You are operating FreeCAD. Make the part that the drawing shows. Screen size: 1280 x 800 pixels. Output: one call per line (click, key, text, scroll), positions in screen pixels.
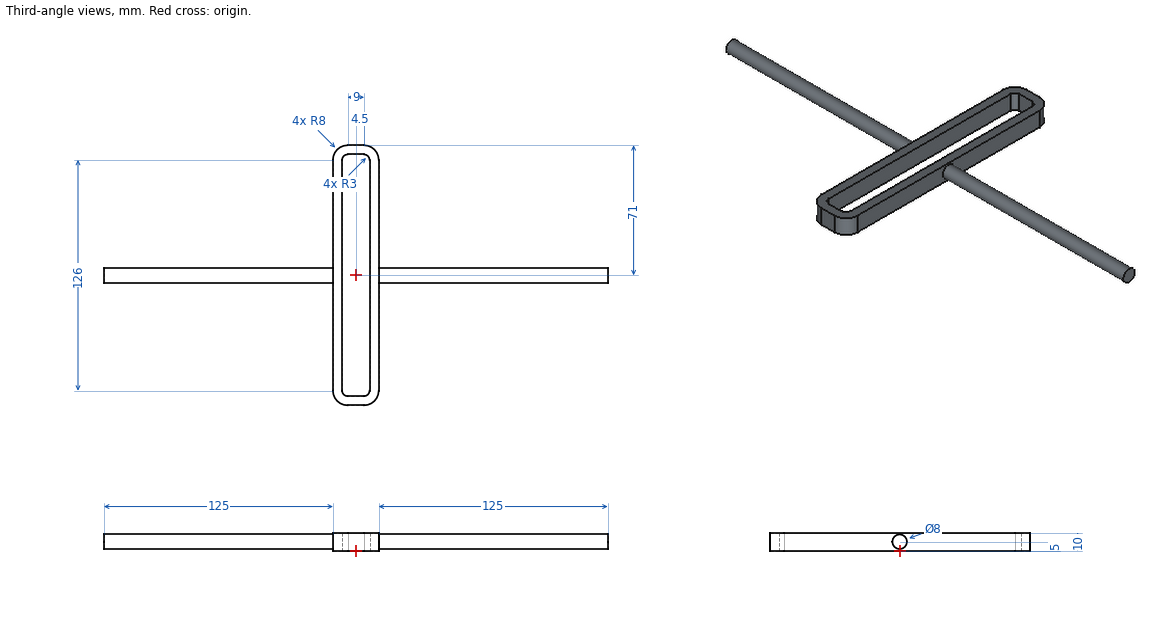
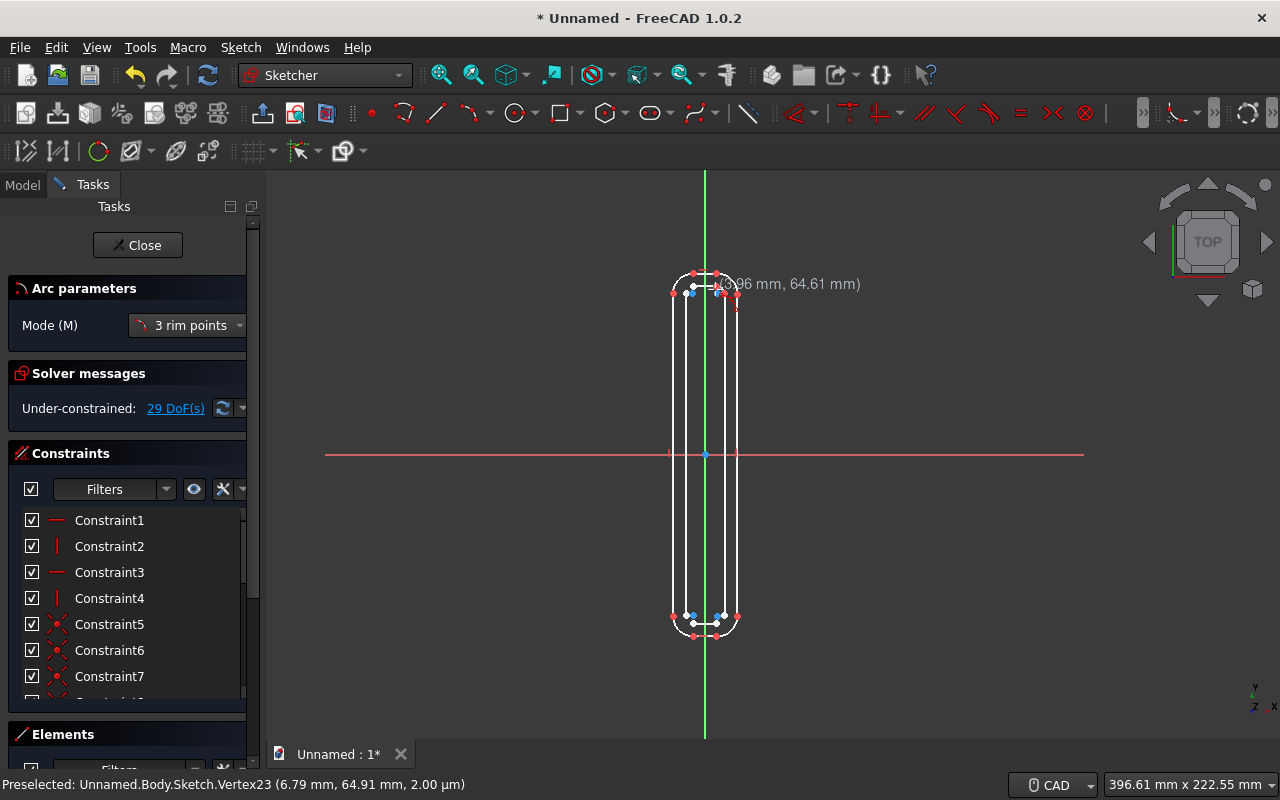
scroll(724, 616, up, 4)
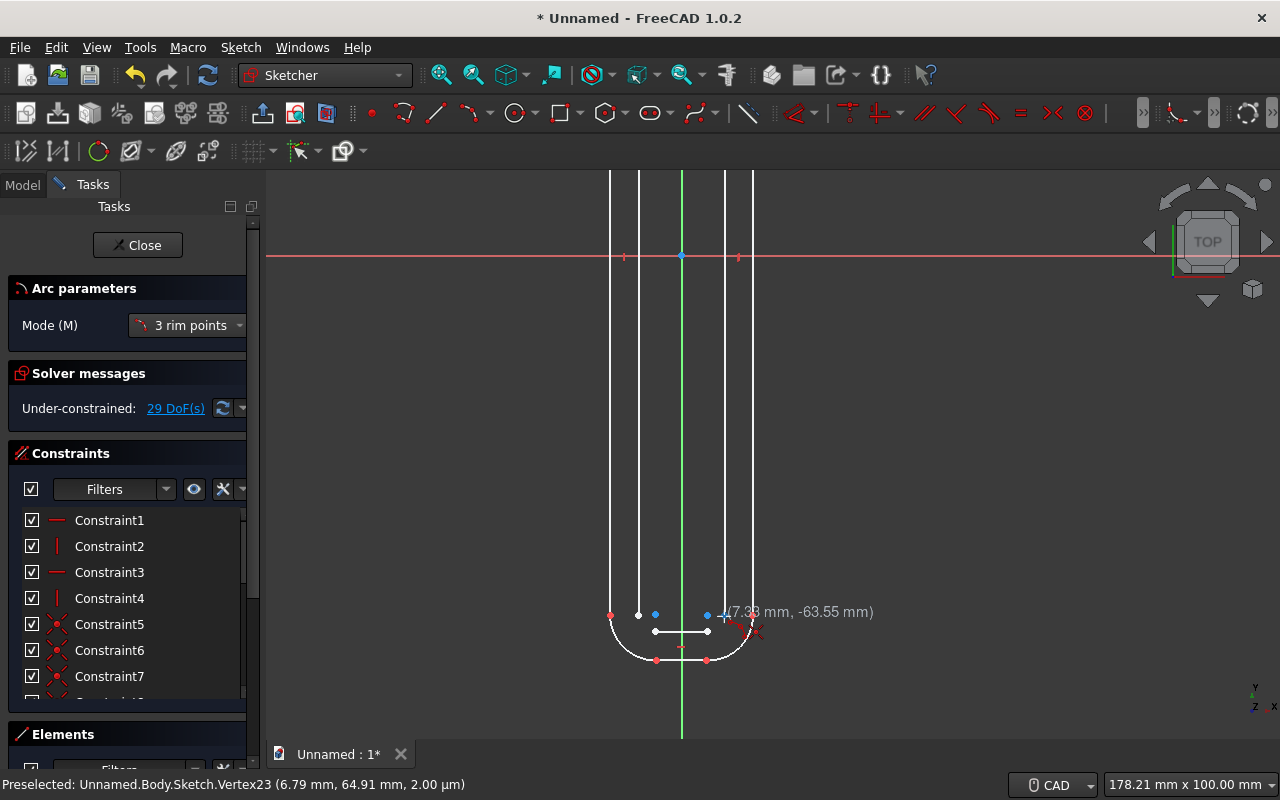
click(725, 615)
click(708, 632)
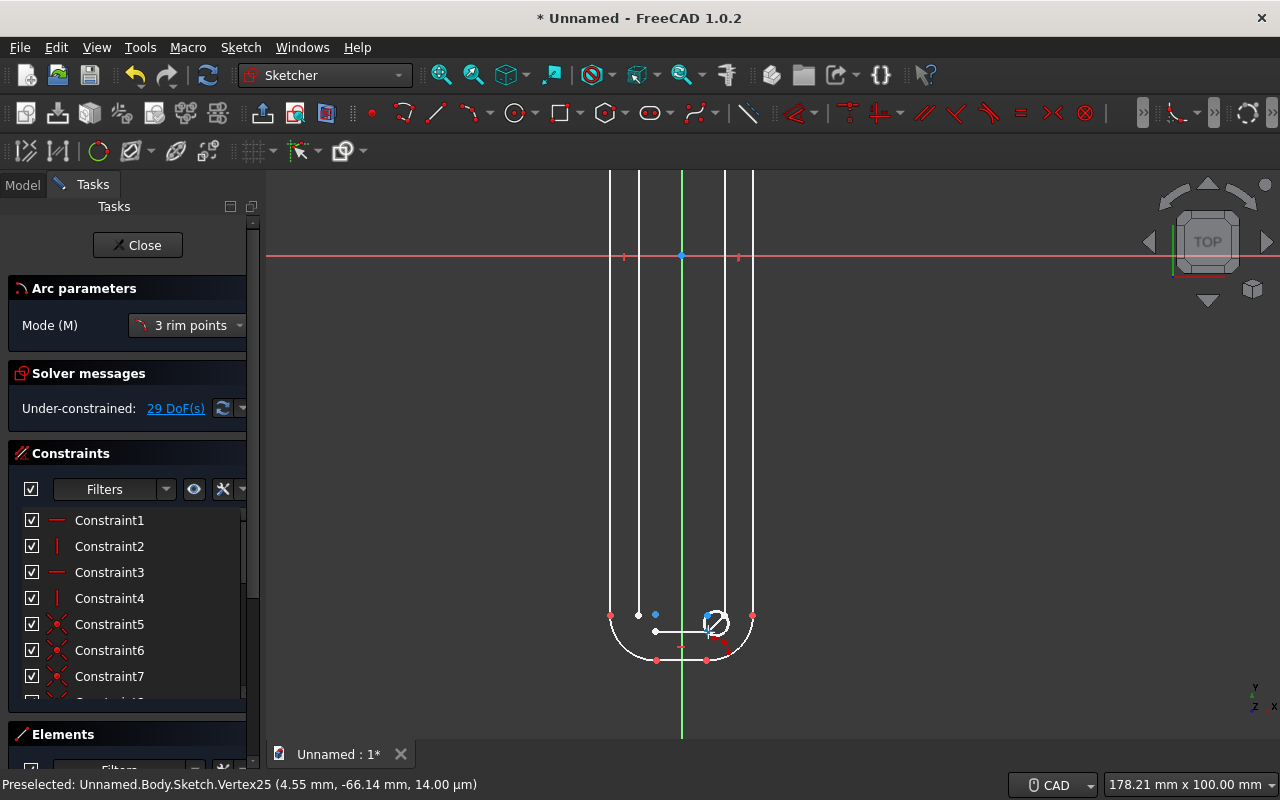
scroll(719, 626, up, 6)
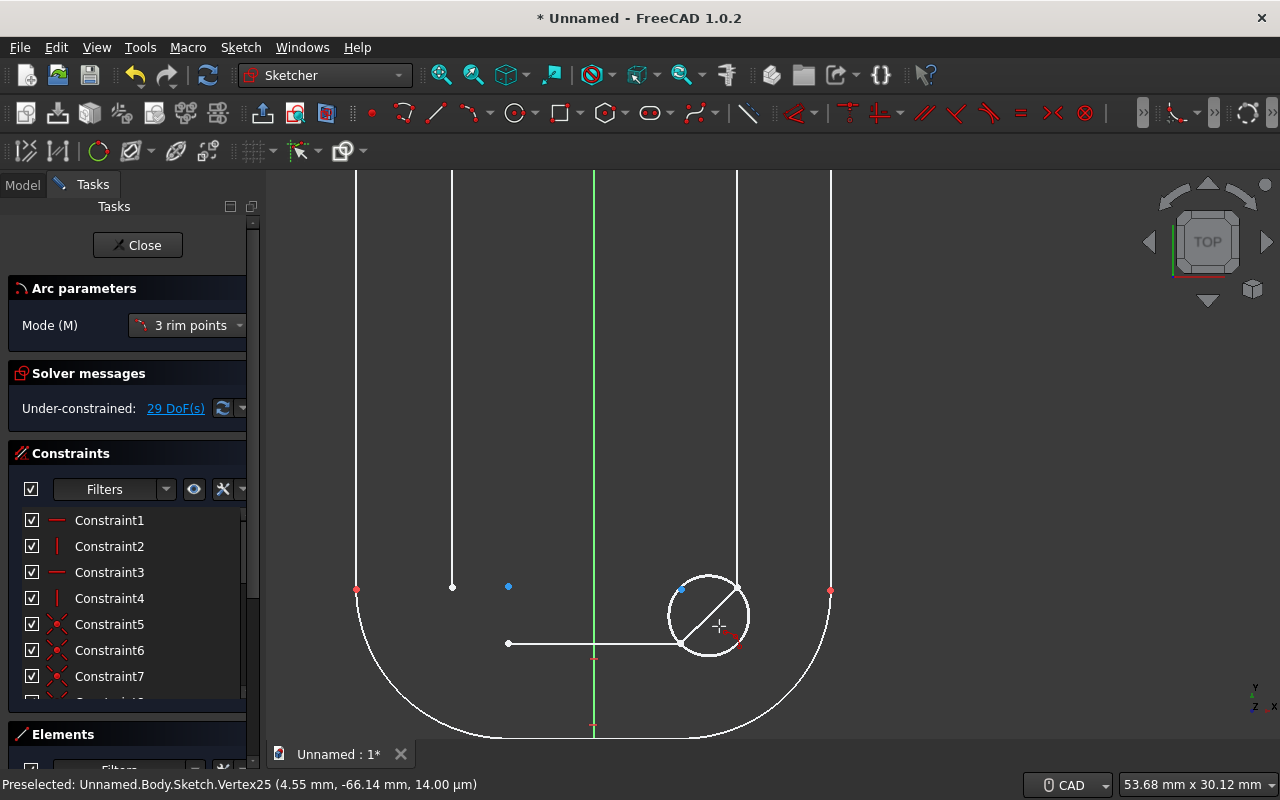
click(719, 625)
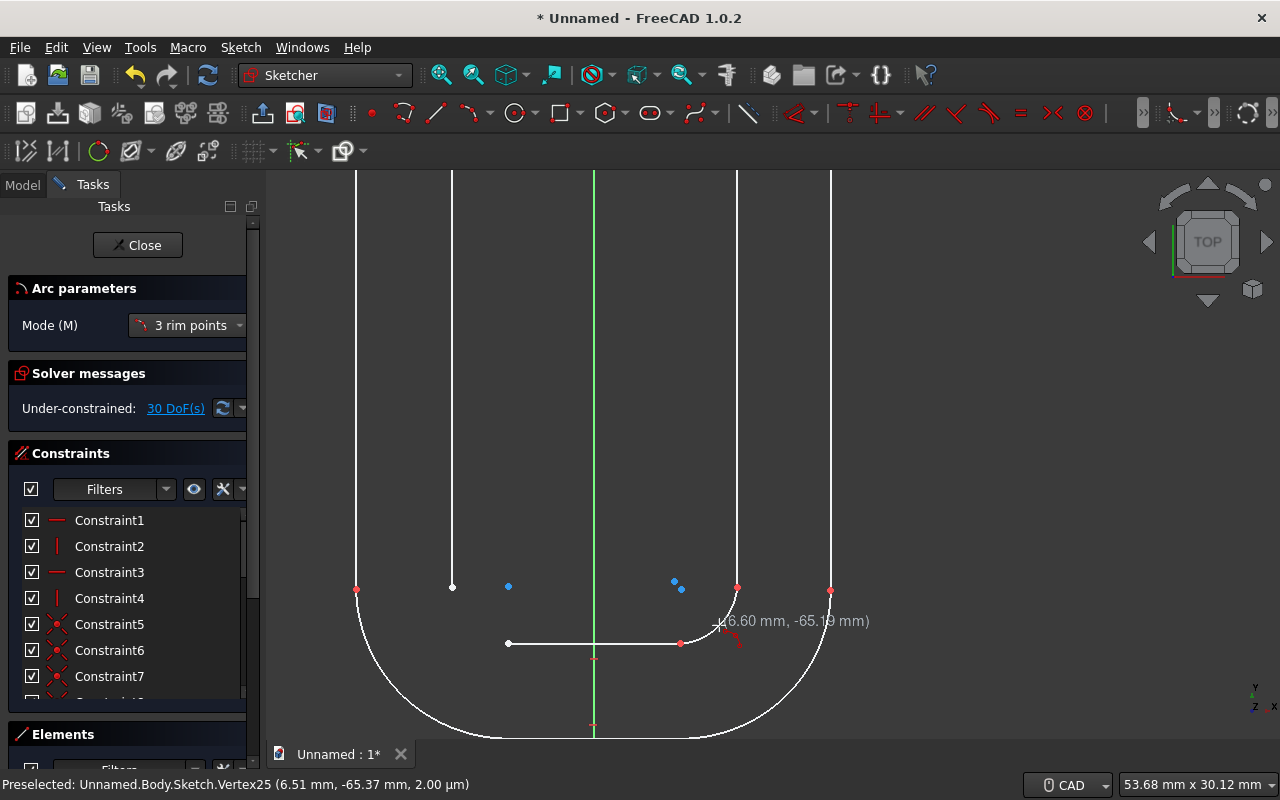
scroll(722, 620, down, 10)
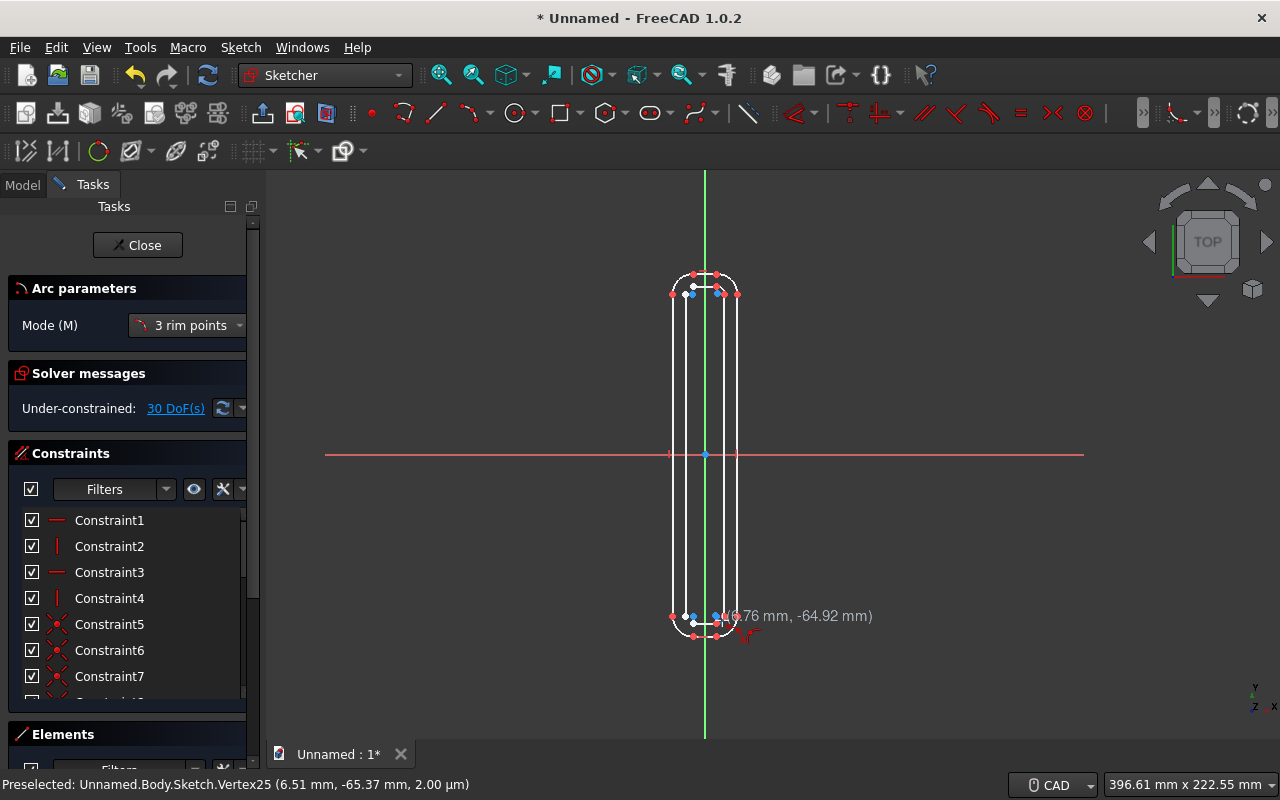
scroll(694, 624, up, 4)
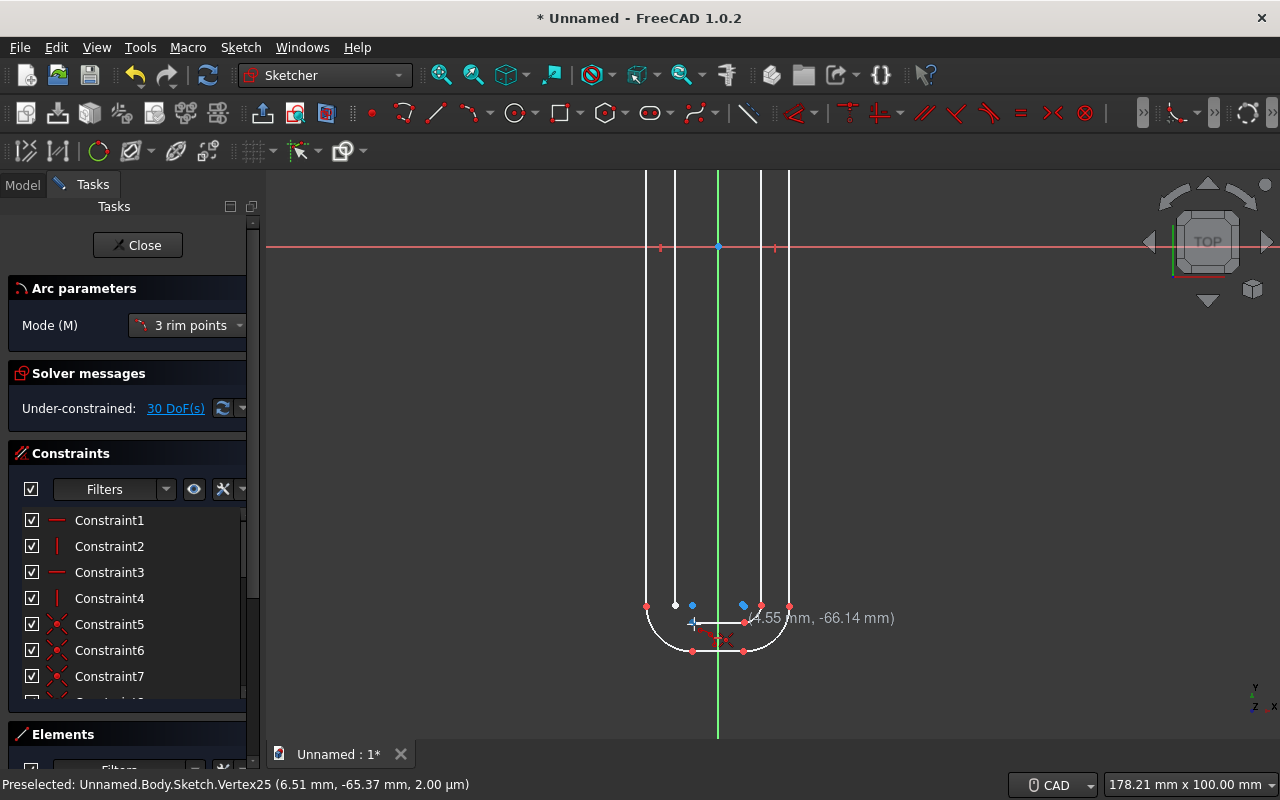
click(692, 623)
click(675, 606)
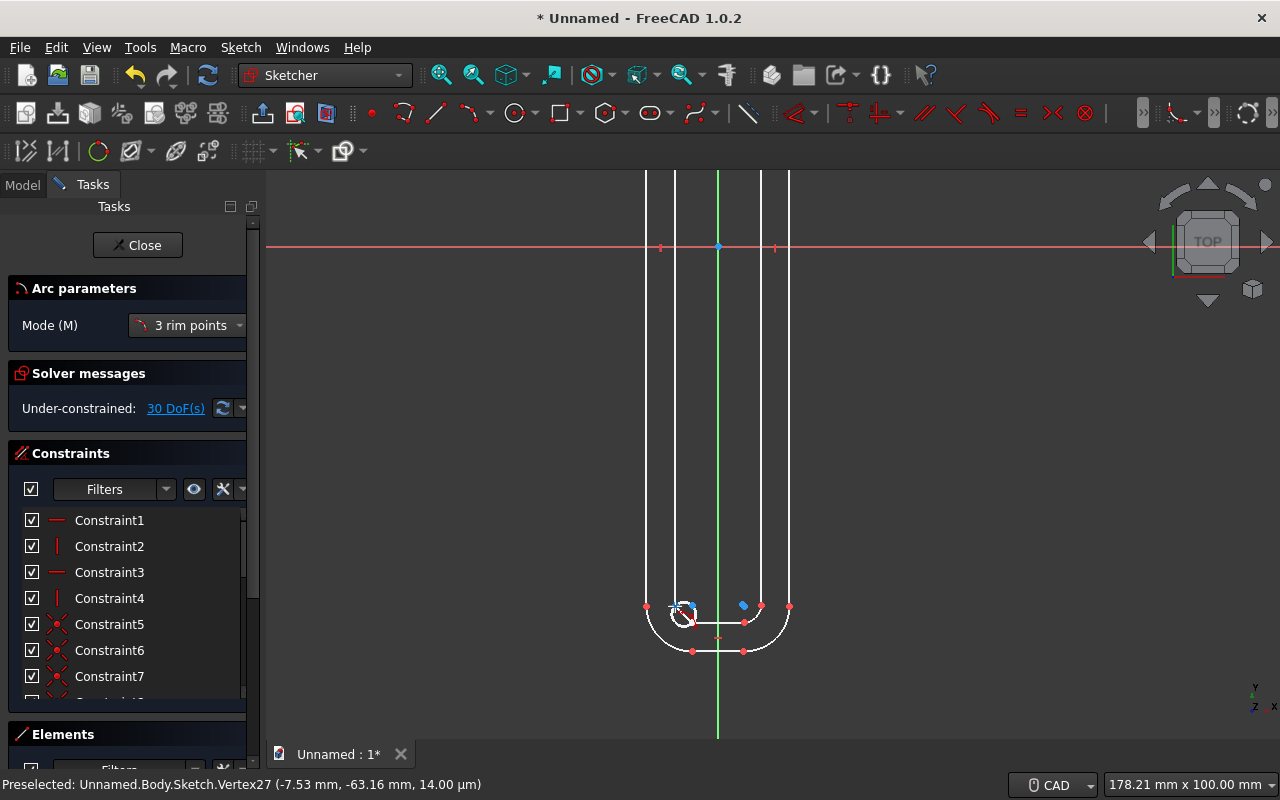
scroll(681, 617, up, 6)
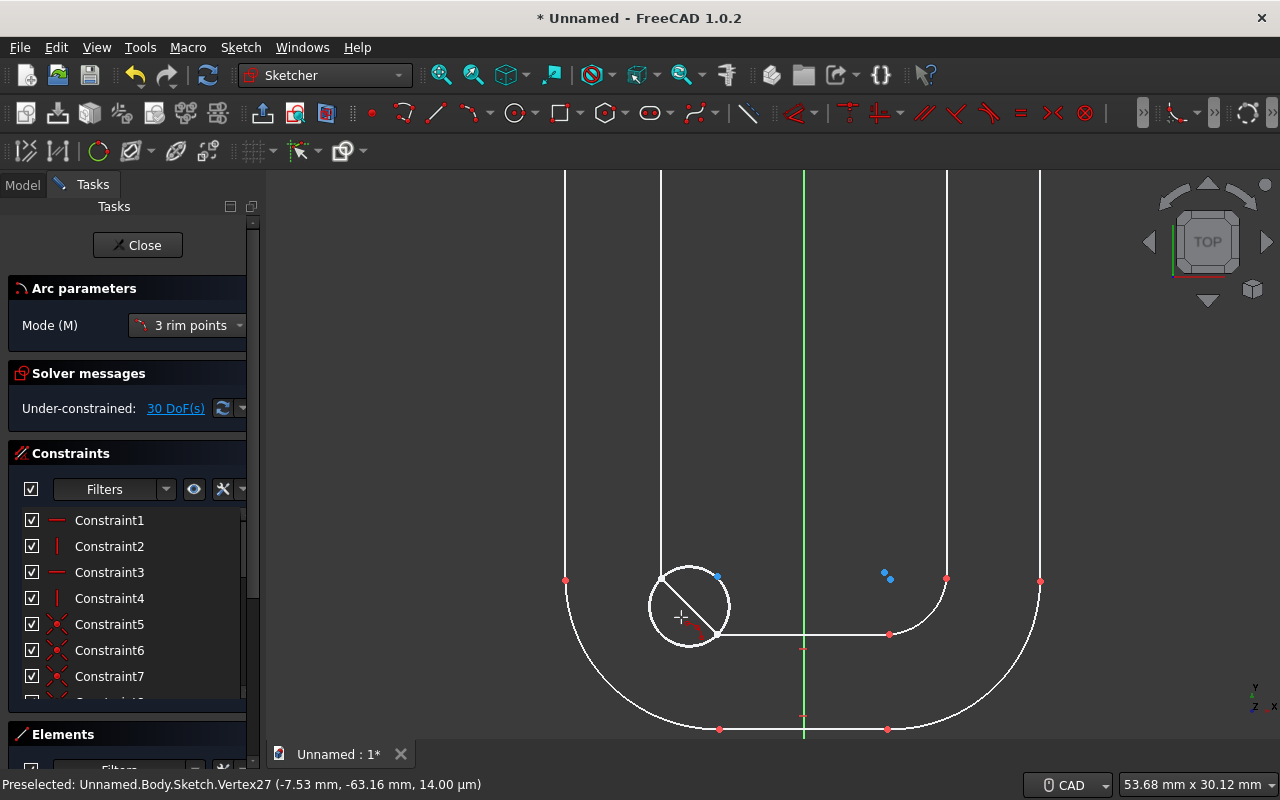
click(678, 615)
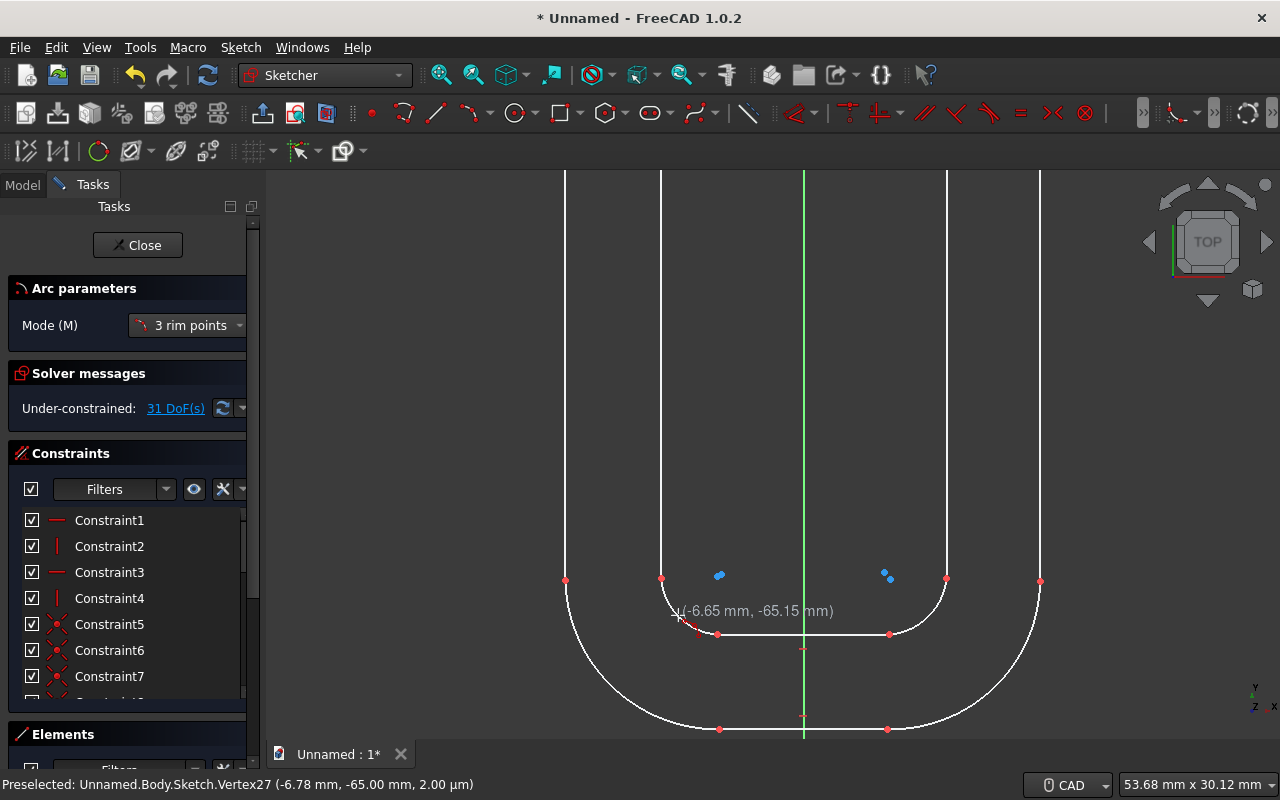
scroll(689, 622, down, 10)